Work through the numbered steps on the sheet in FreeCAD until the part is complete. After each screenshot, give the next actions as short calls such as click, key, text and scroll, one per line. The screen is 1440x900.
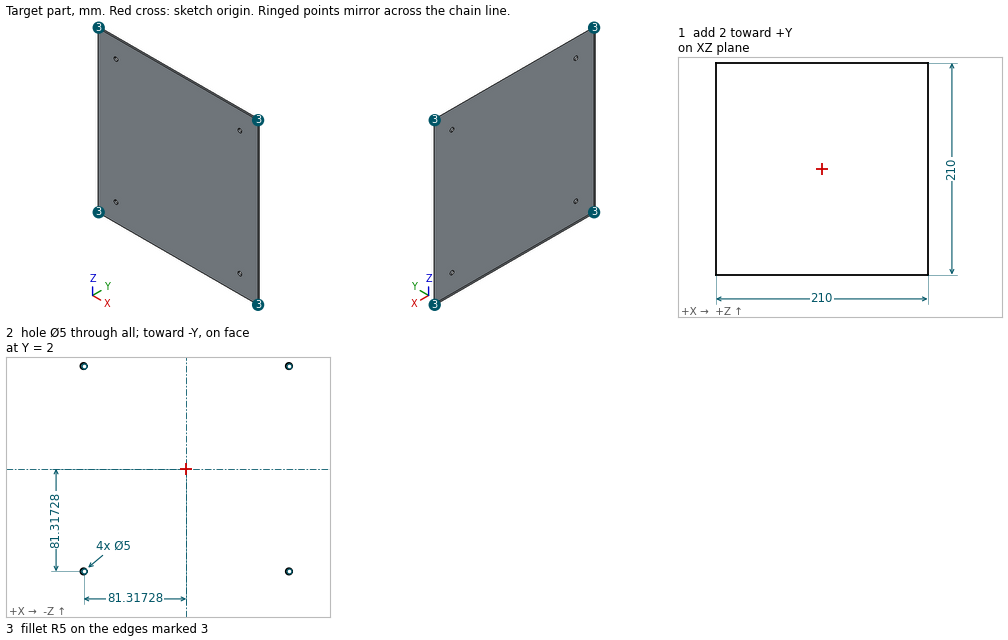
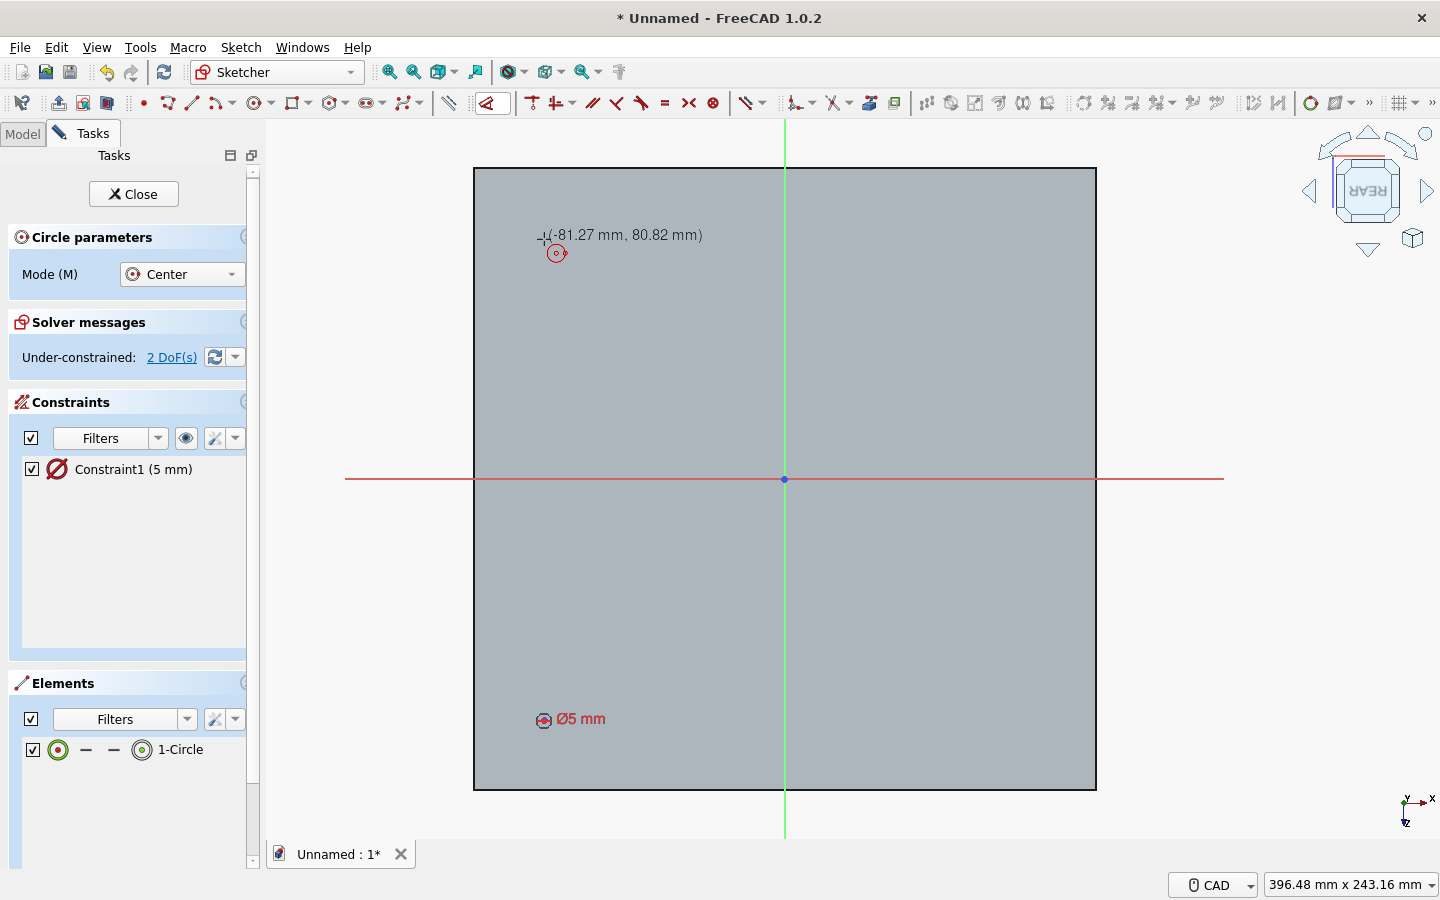
click(544, 239)
move(549, 233)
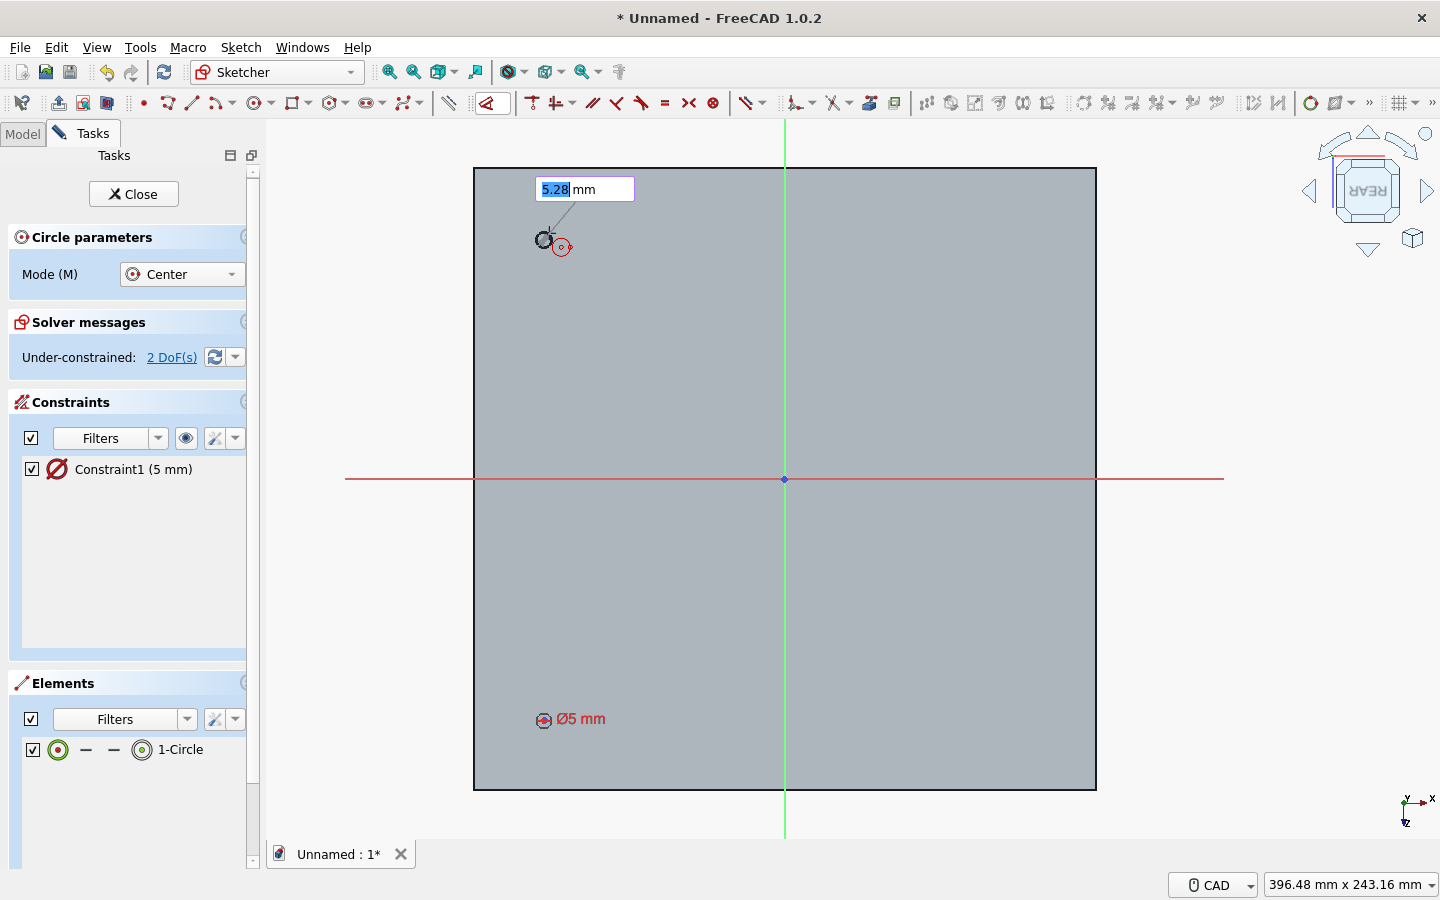
text(5)
key(Return)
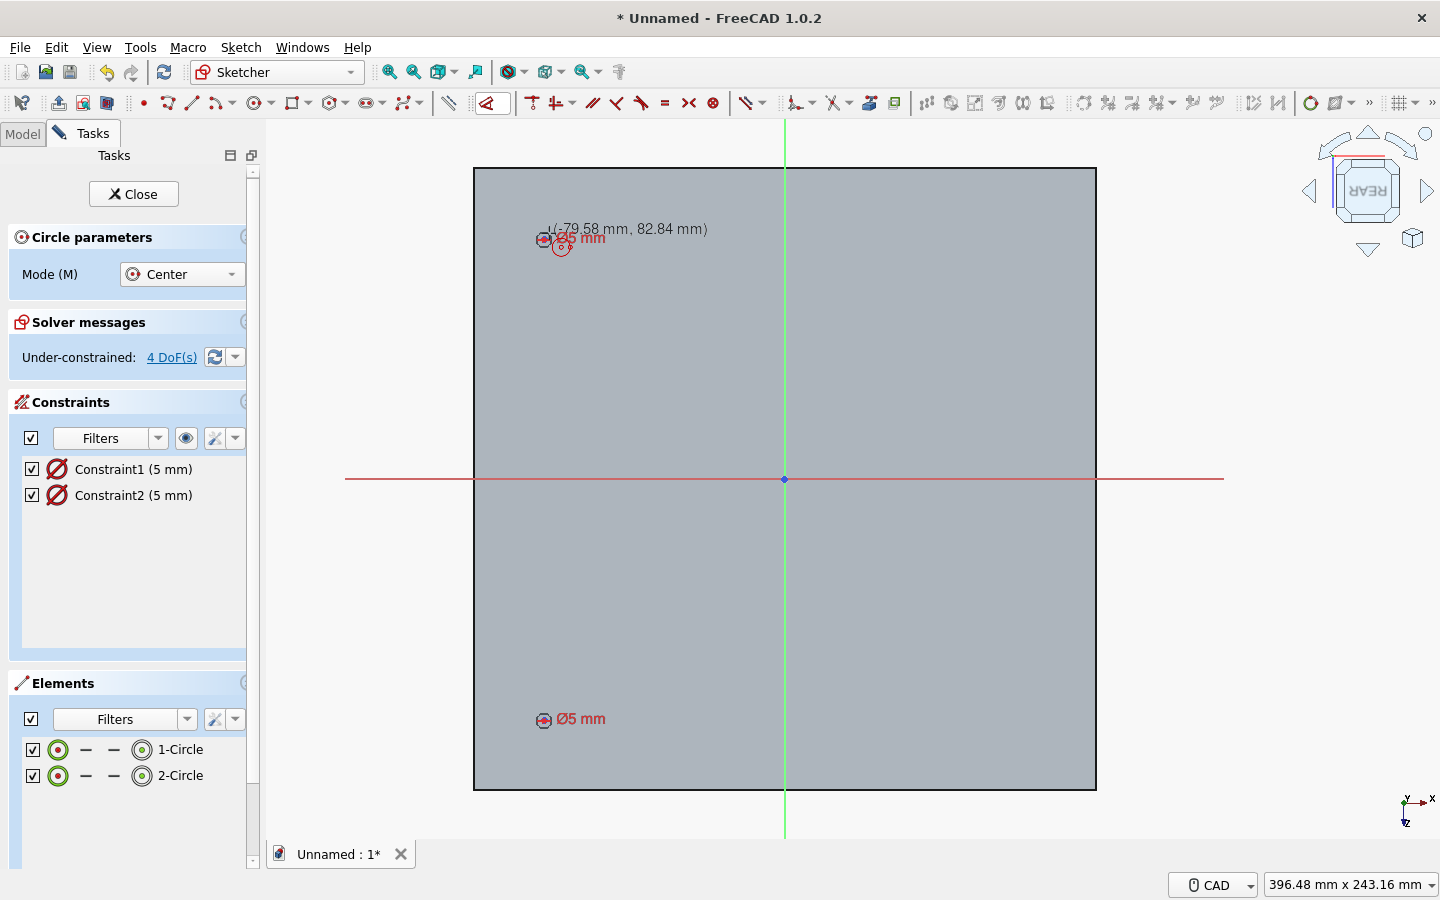
scroll(1025, 239, up, 6)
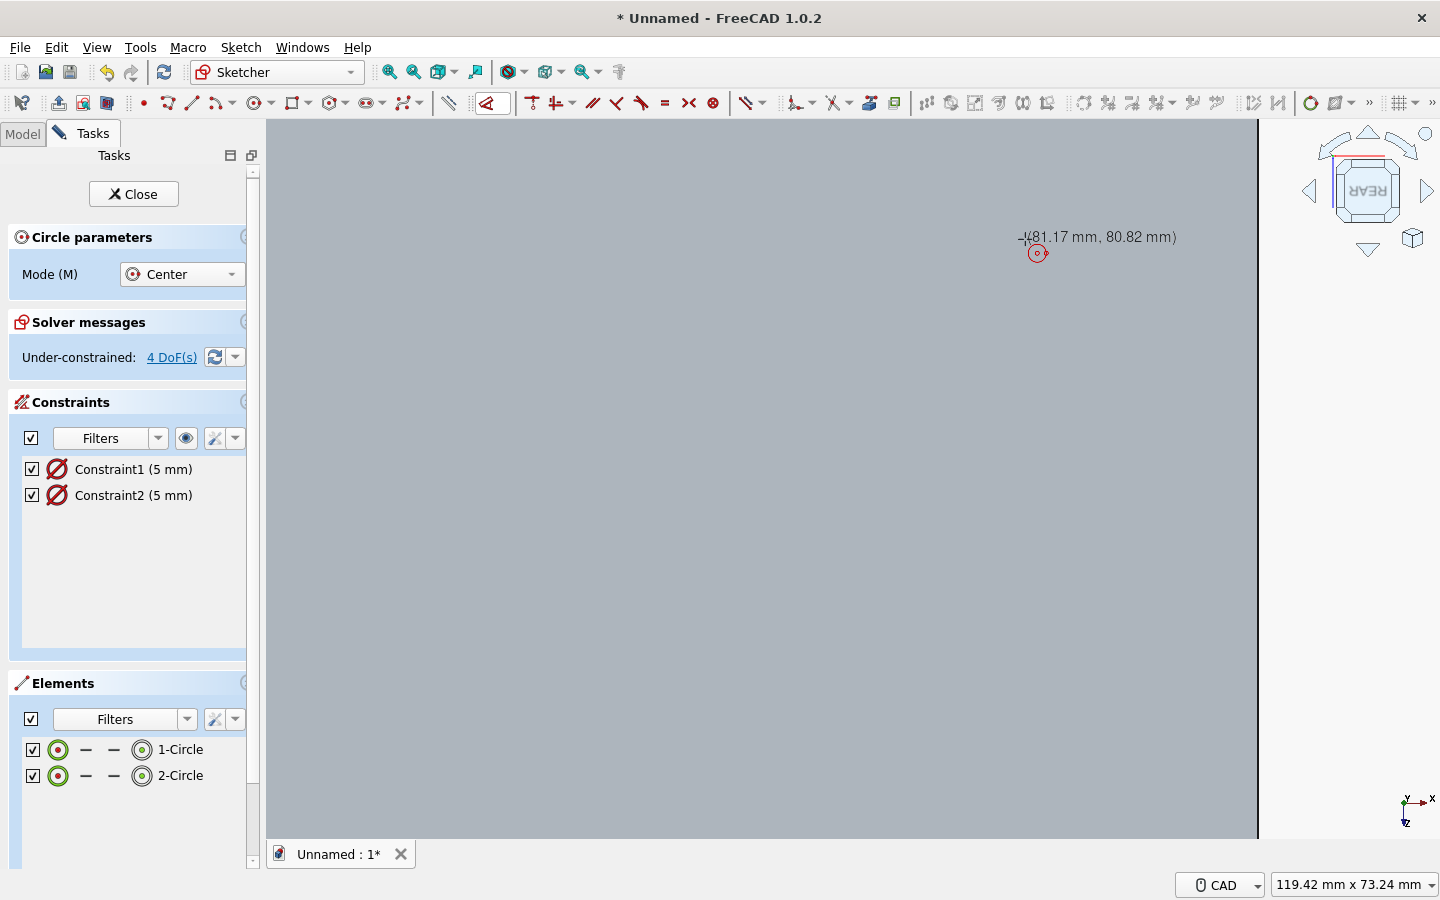
scroll(1025, 239, down, 6)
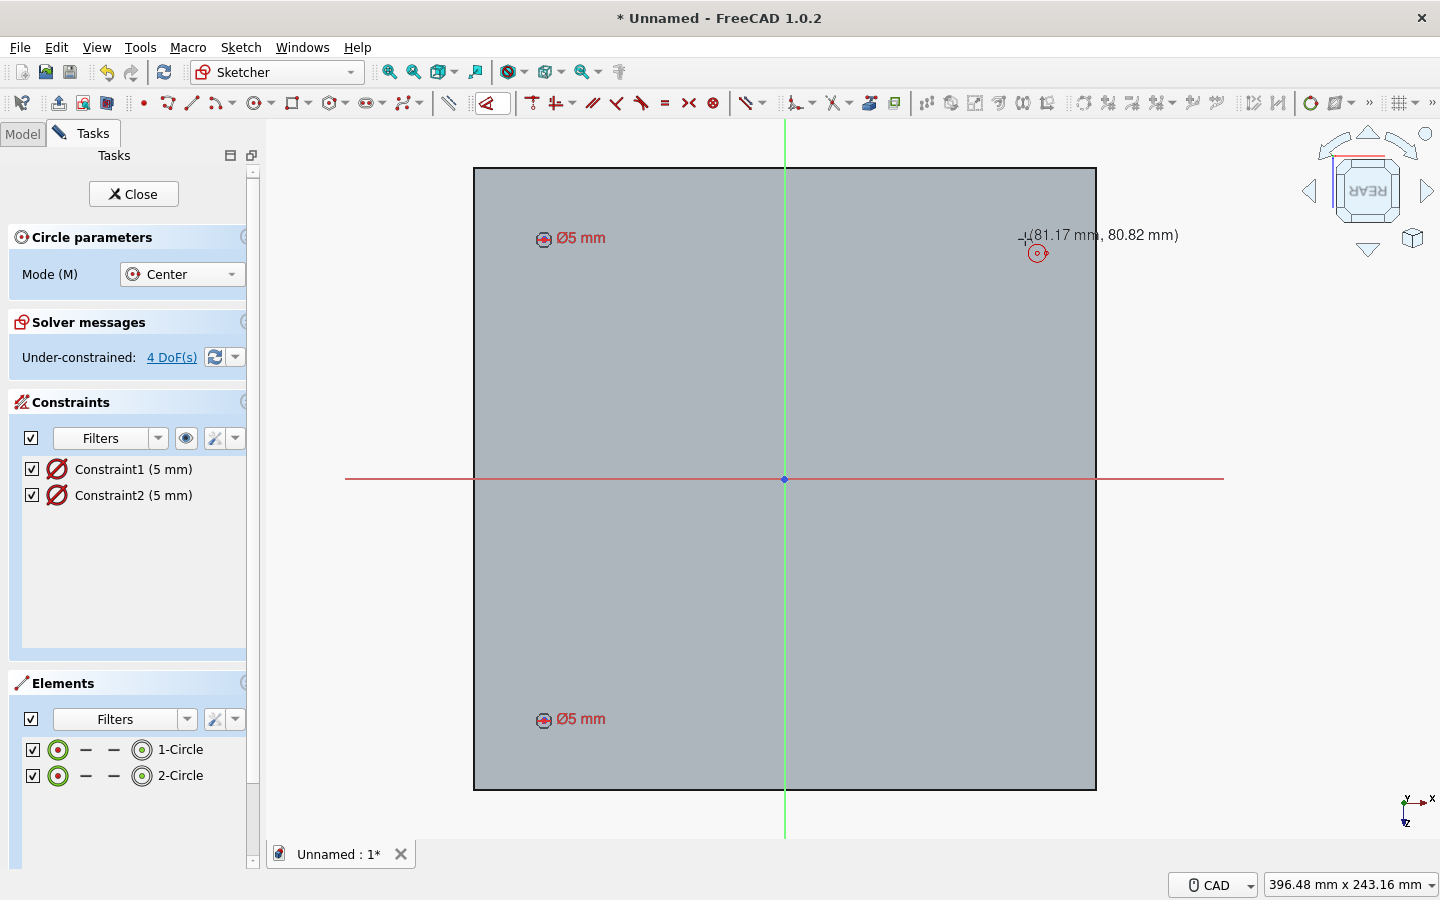
click(1025, 239)
move(1031, 233)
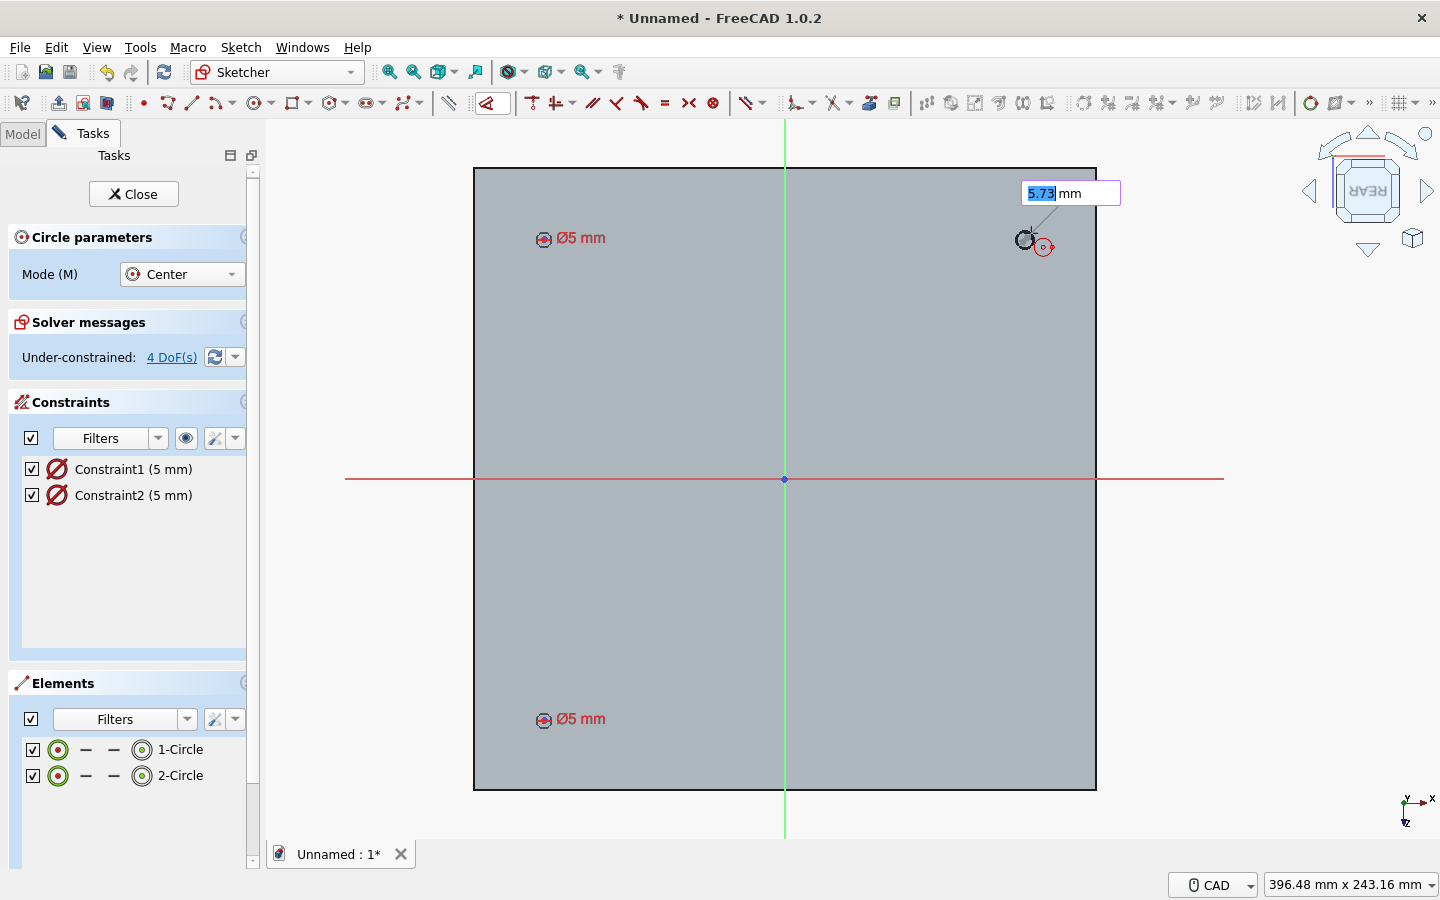
text(5)
key(Return)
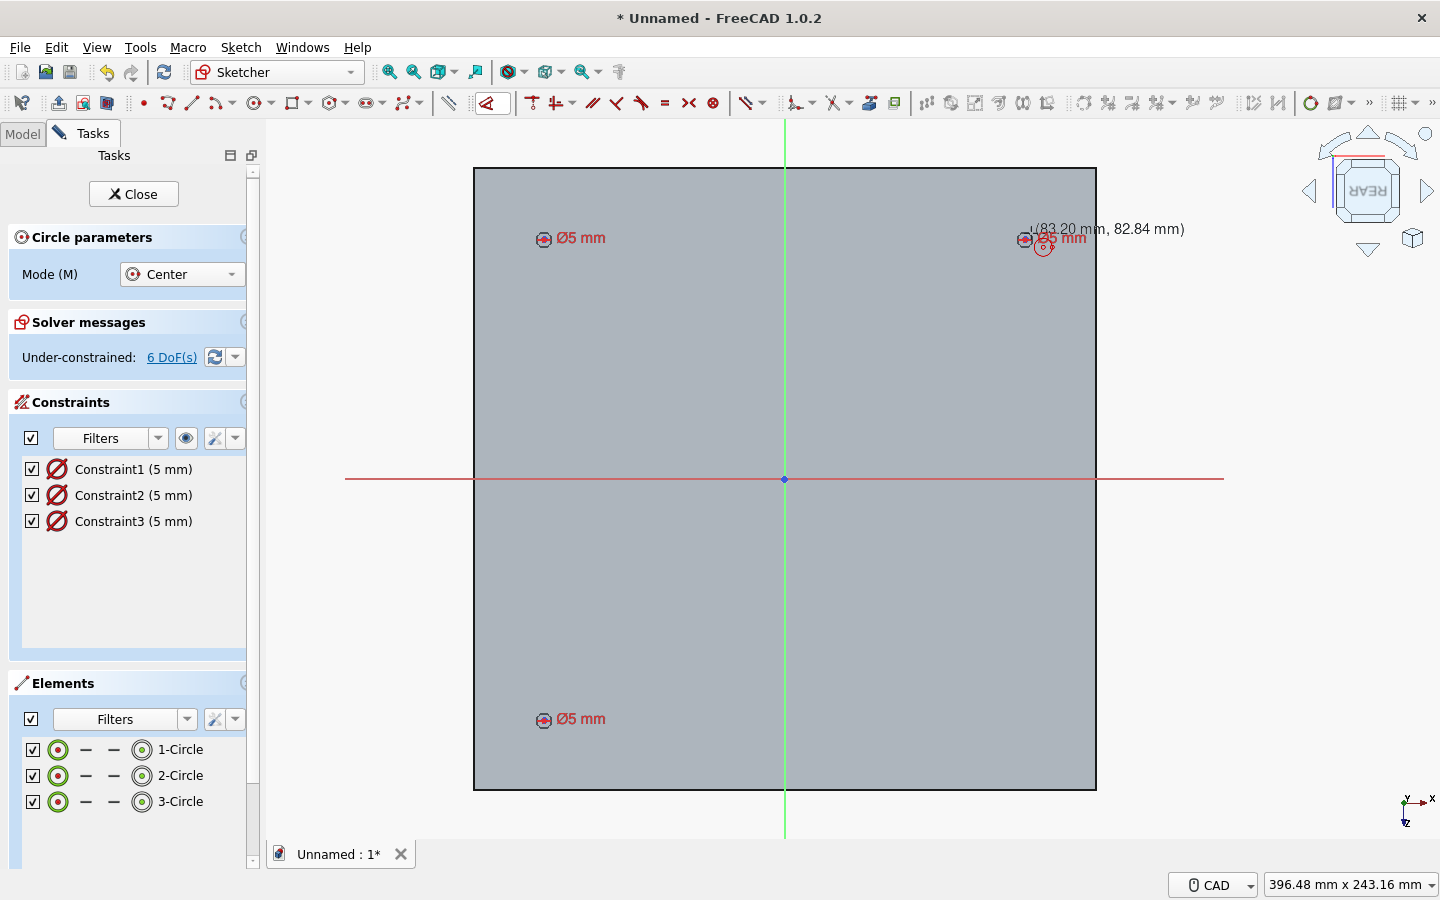
scroll(1025, 720, up, 6)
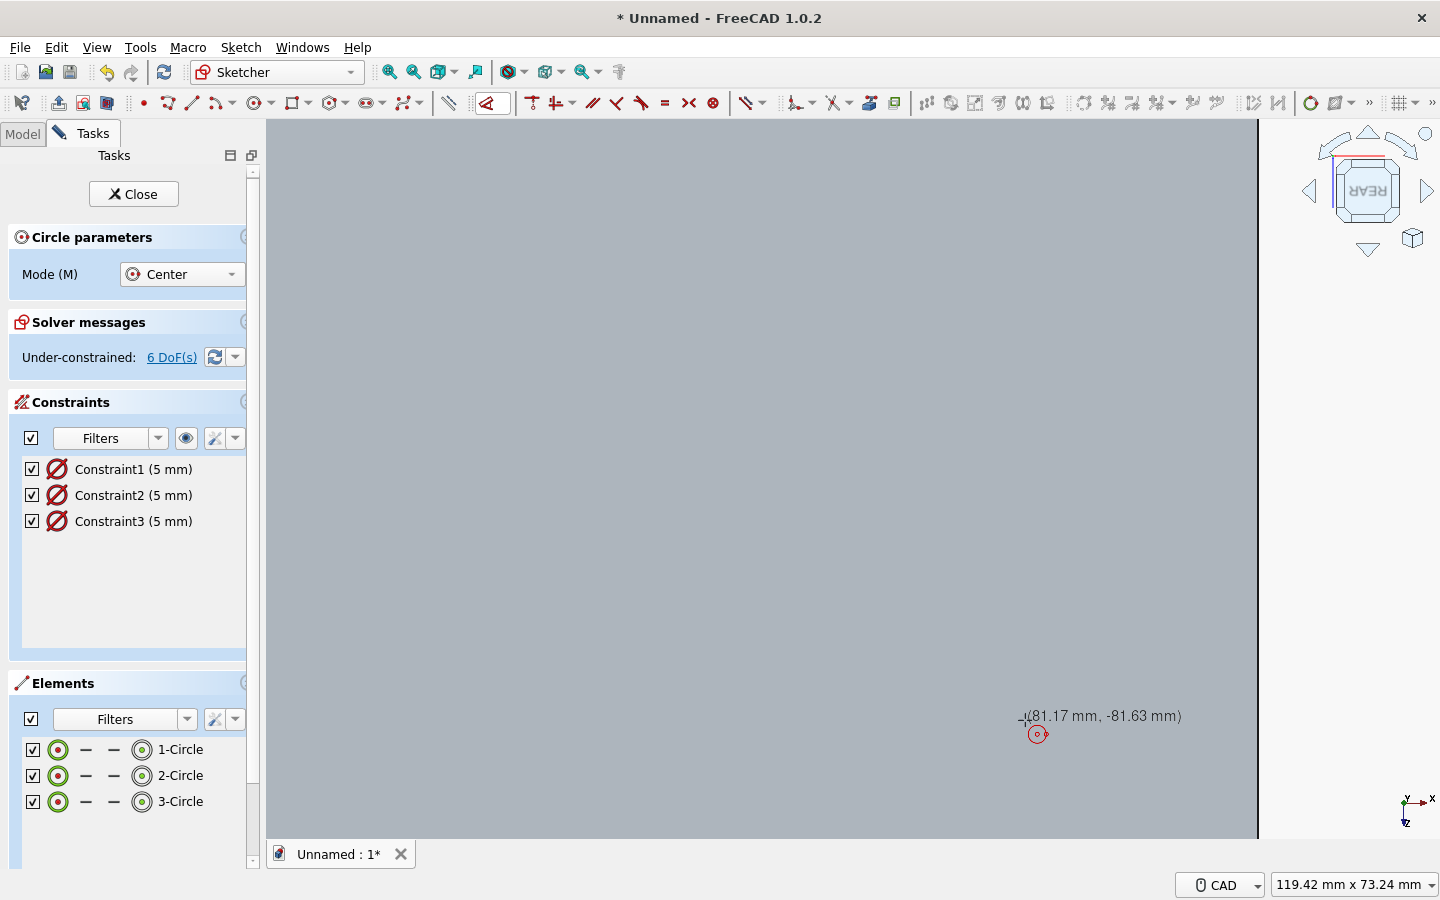
scroll(1025, 720, down, 6)